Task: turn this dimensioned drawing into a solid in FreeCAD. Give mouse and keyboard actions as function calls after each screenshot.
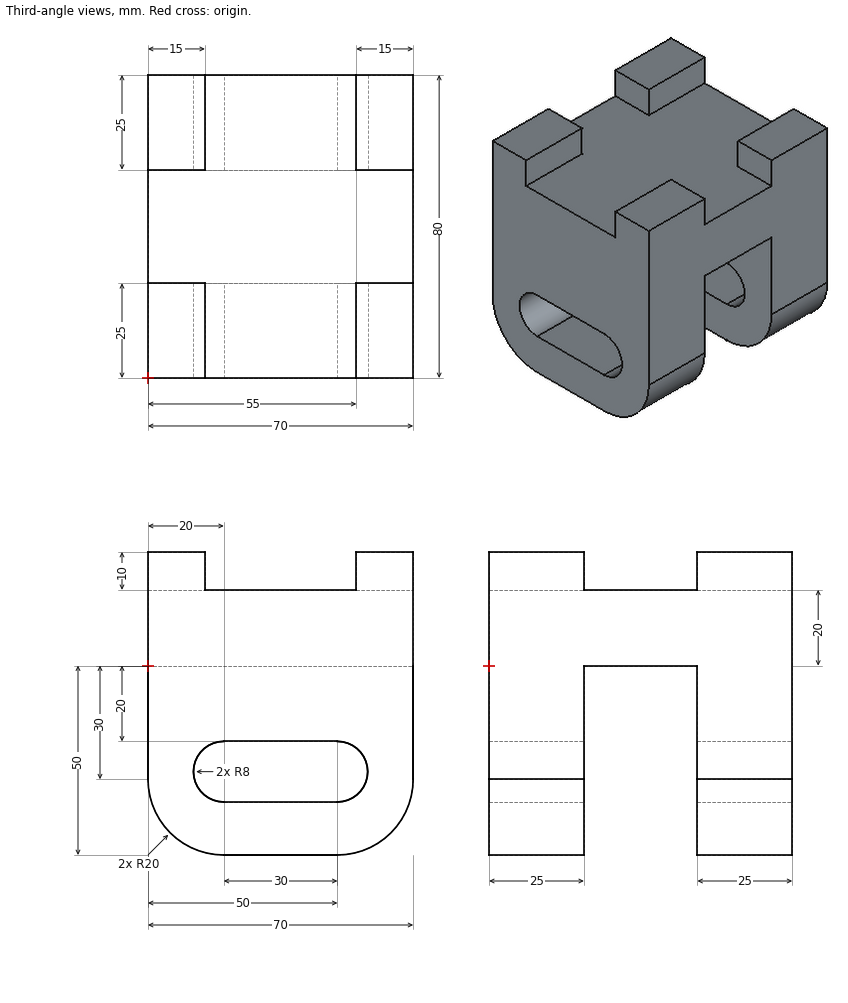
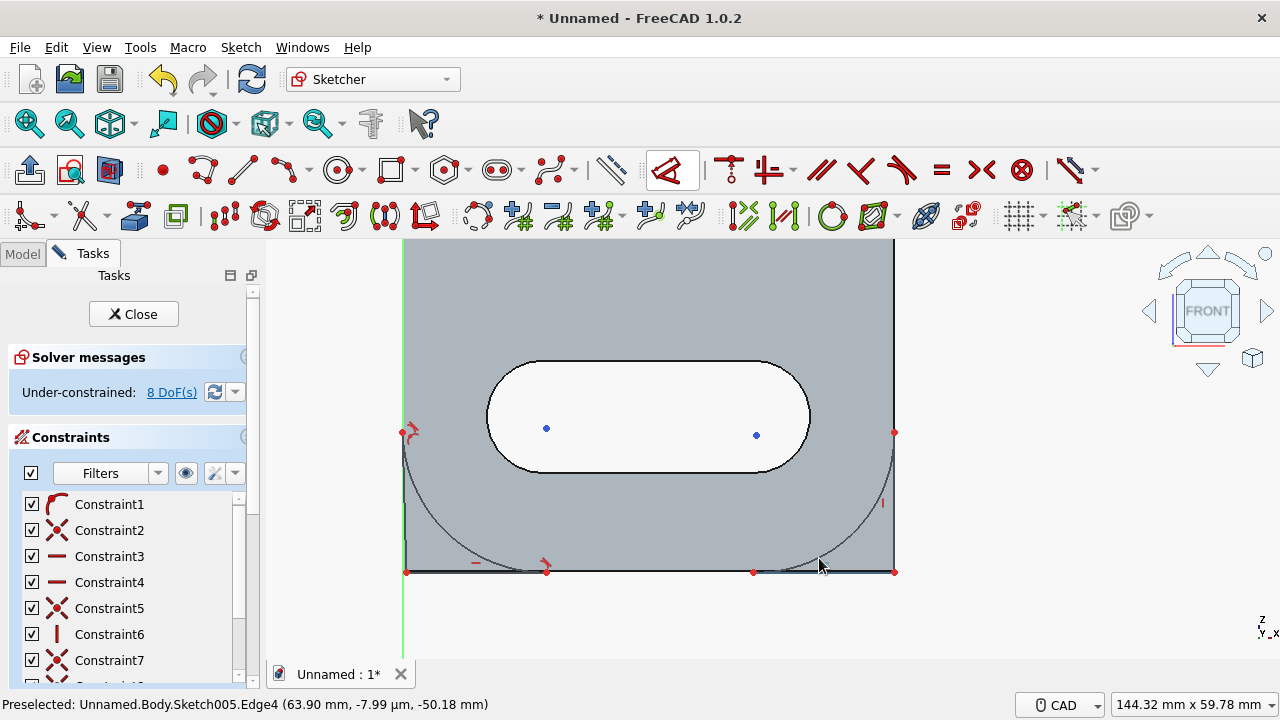
click(818, 558)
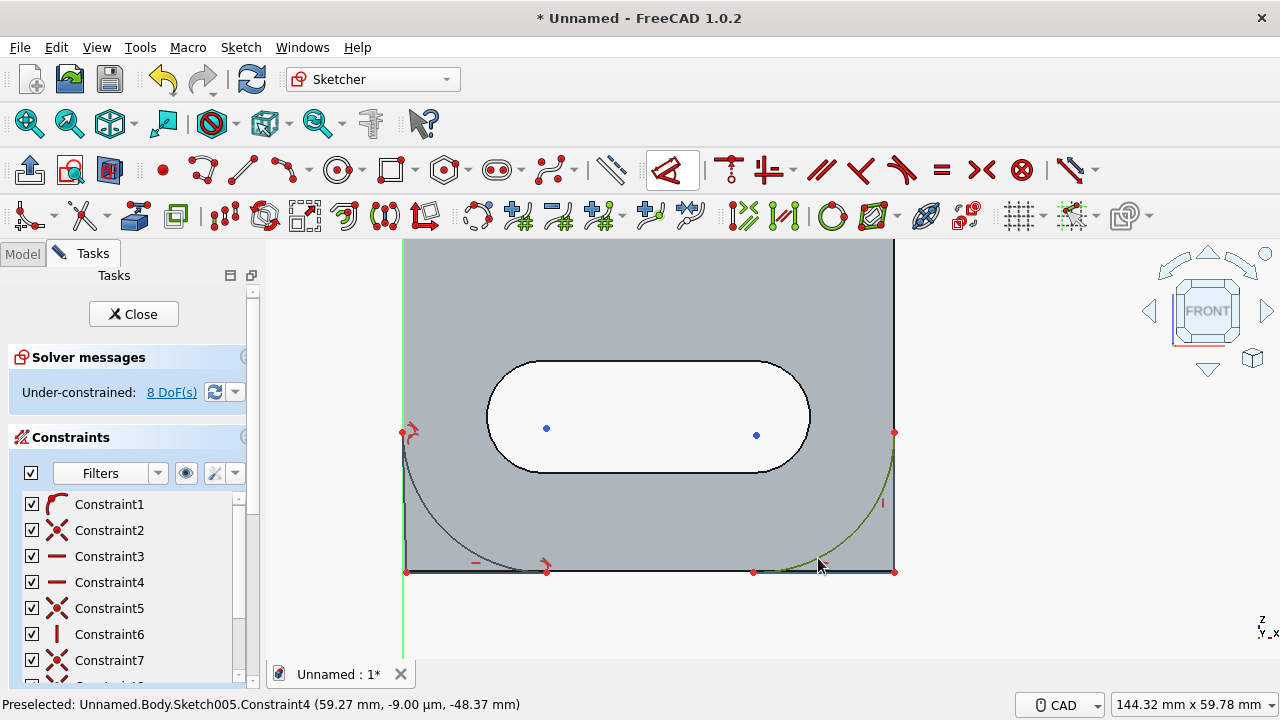
click(902, 170)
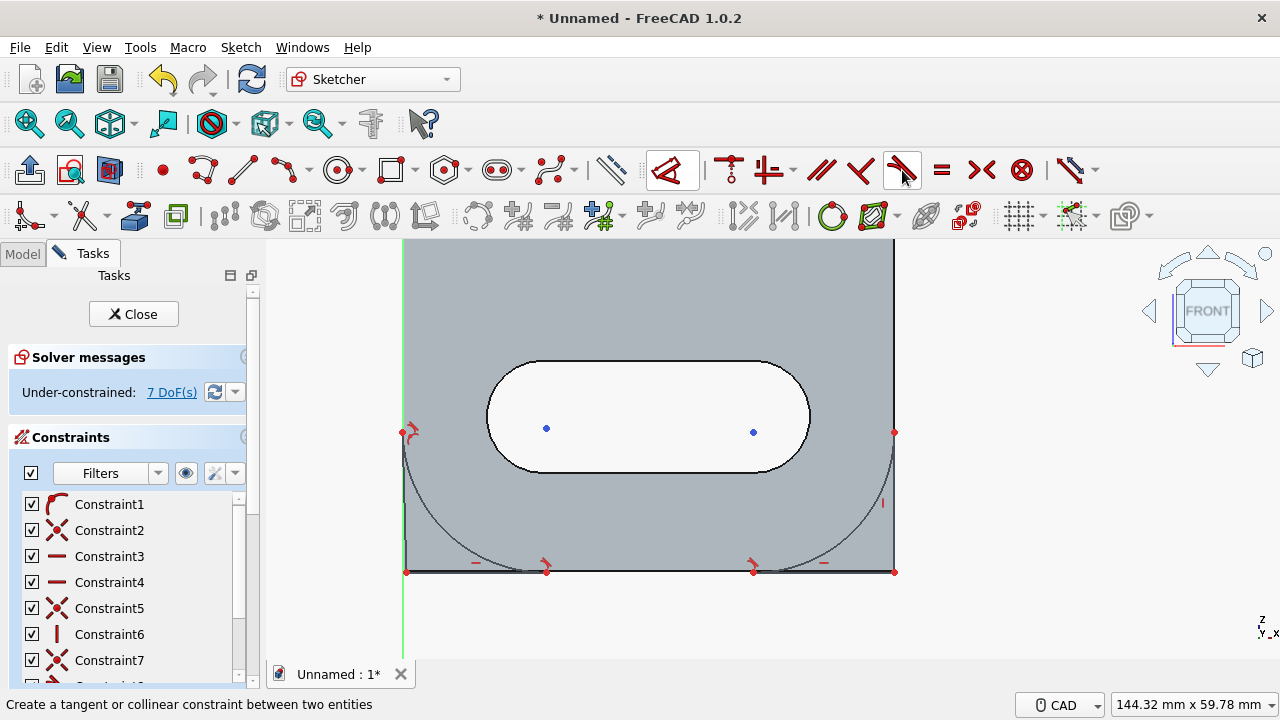
click(894, 531)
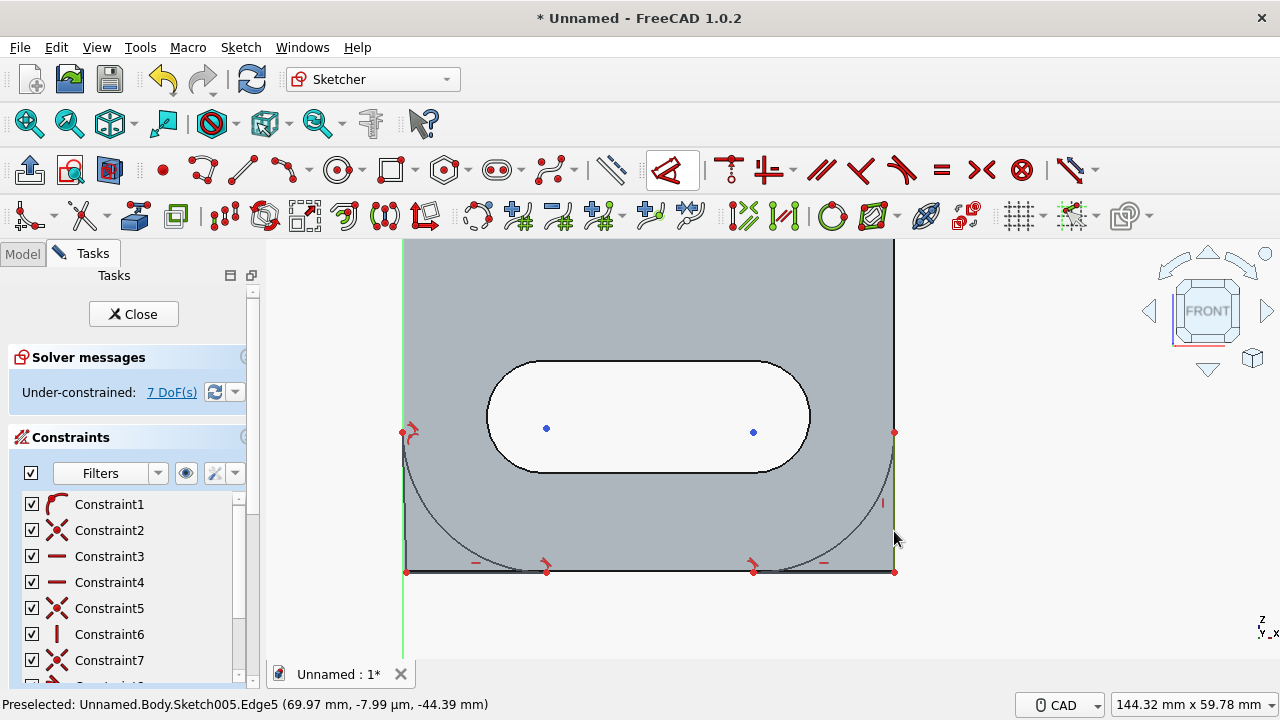
click(818, 557)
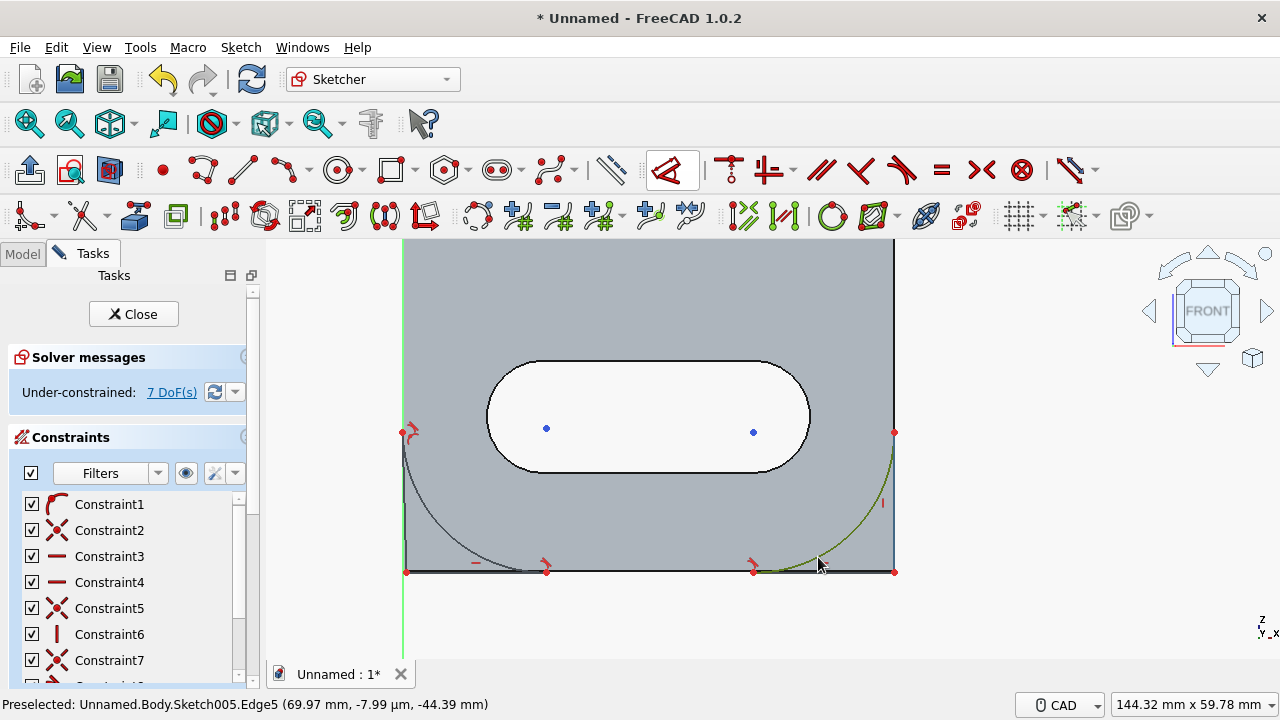
click(902, 170)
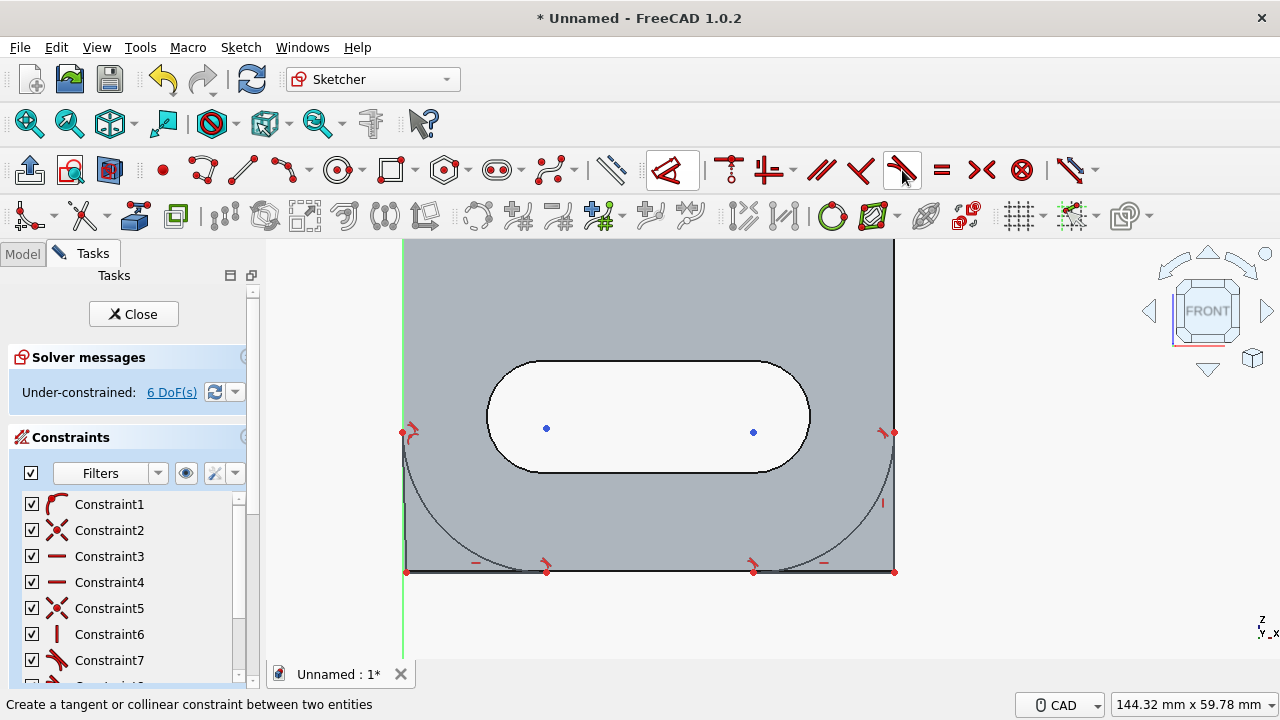
click(405, 531)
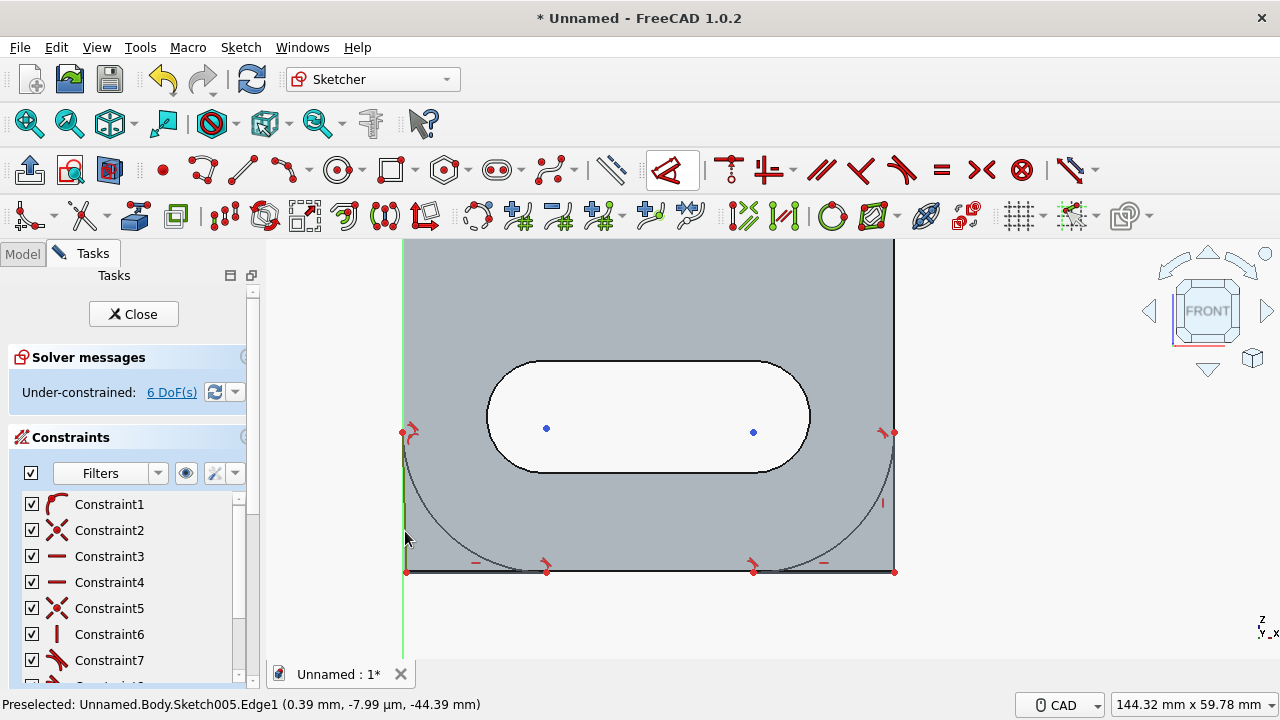
click(796, 170)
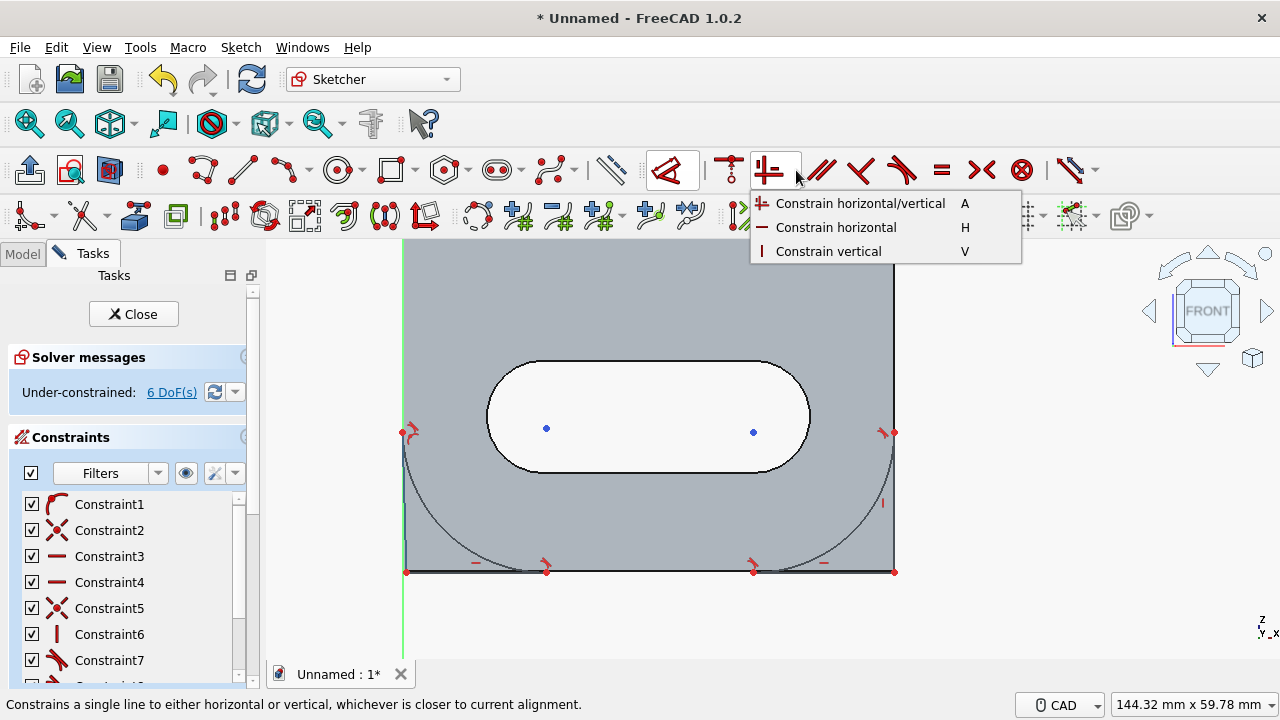
click(886, 251)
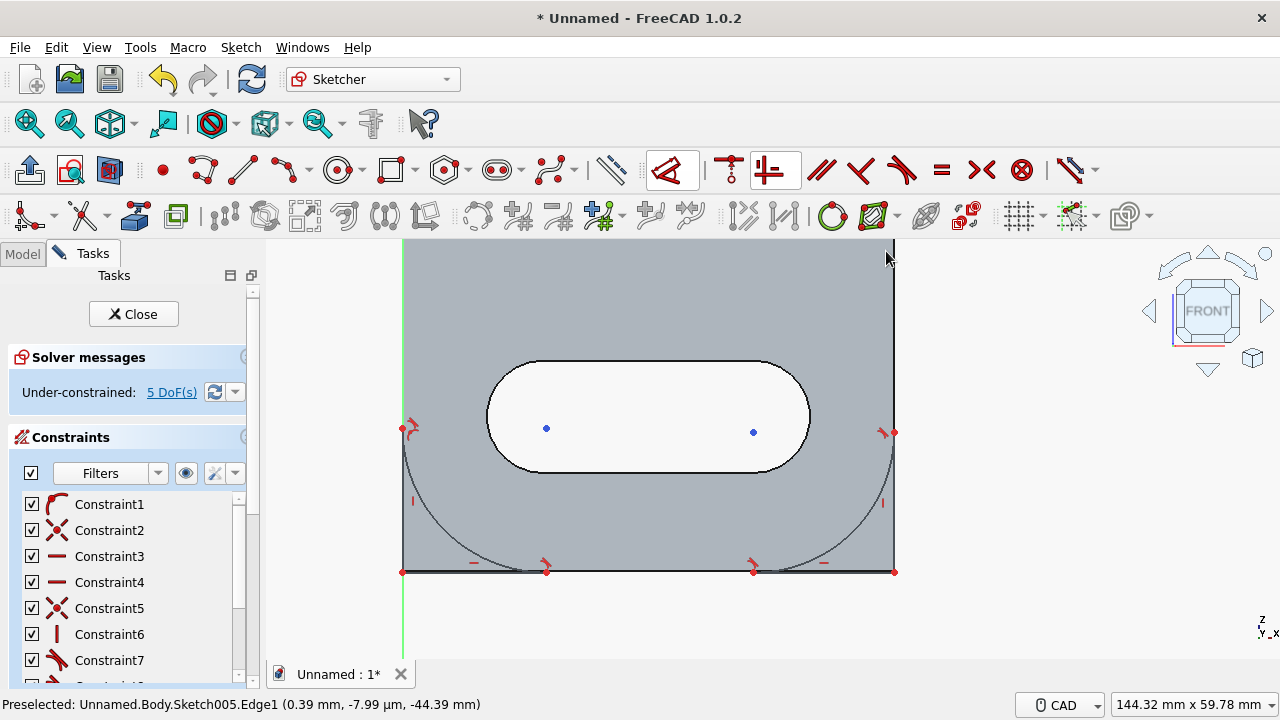
click(481, 557)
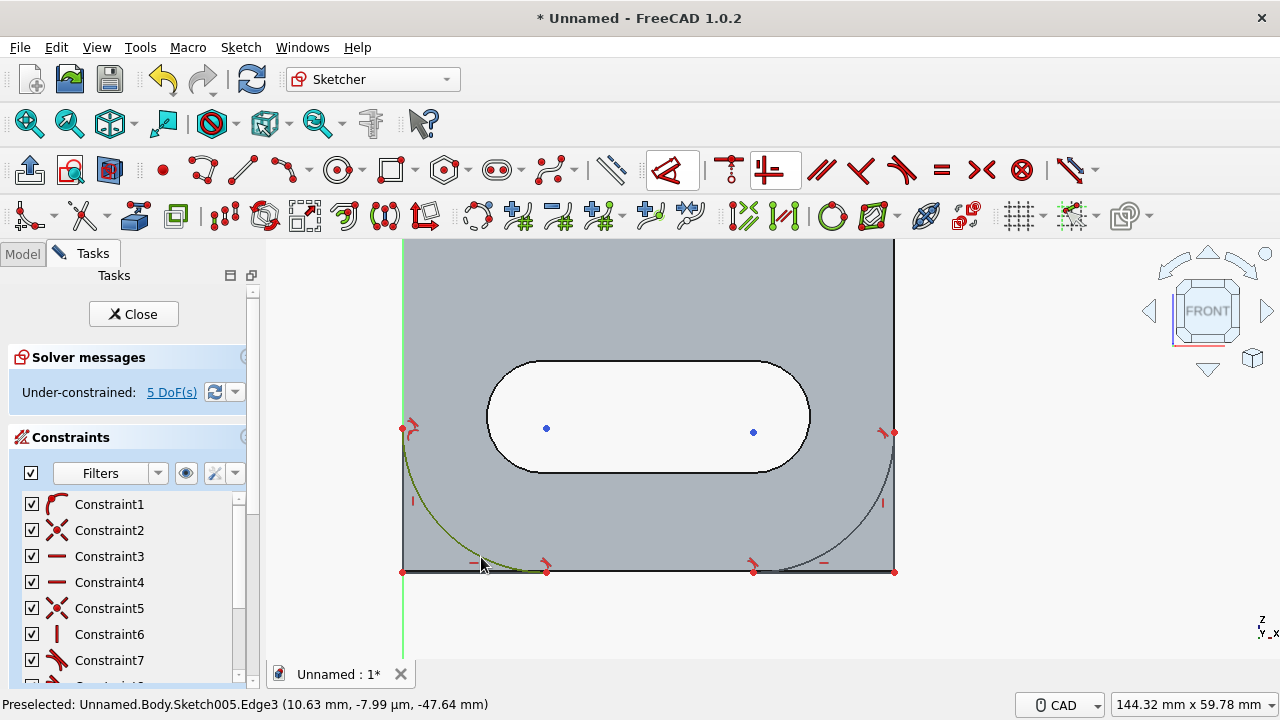
click(818, 557)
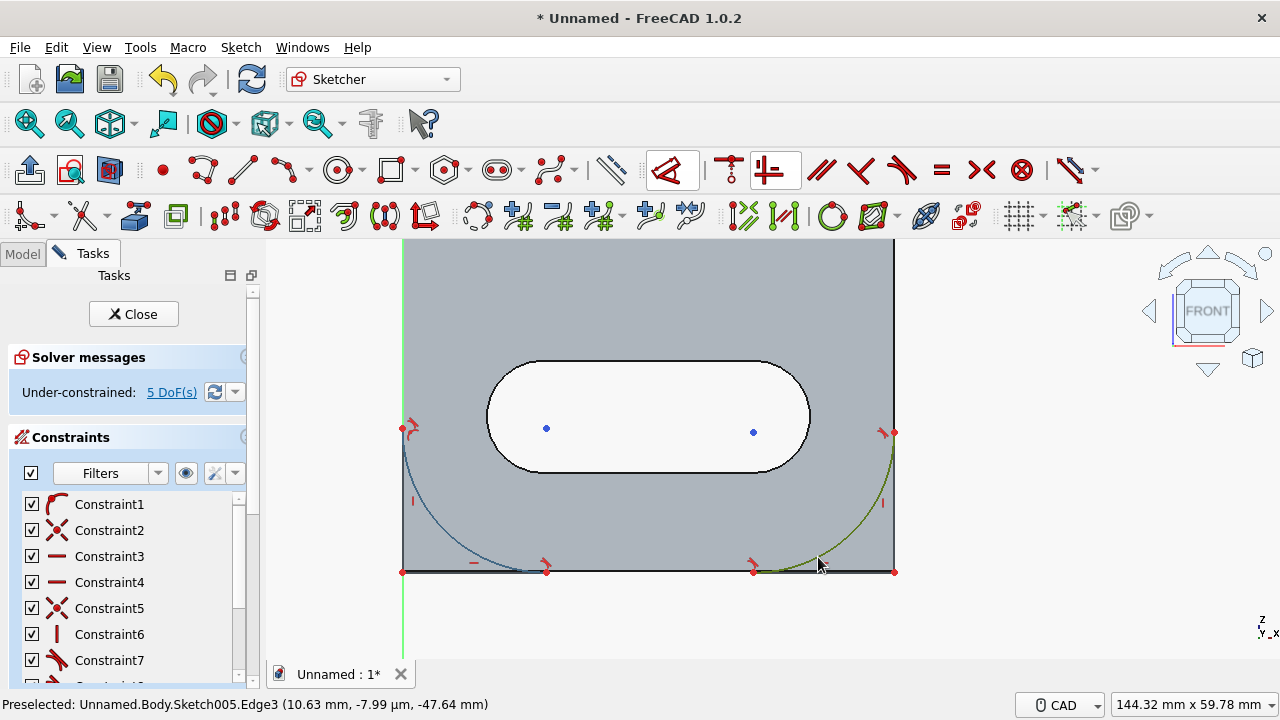
key(e)